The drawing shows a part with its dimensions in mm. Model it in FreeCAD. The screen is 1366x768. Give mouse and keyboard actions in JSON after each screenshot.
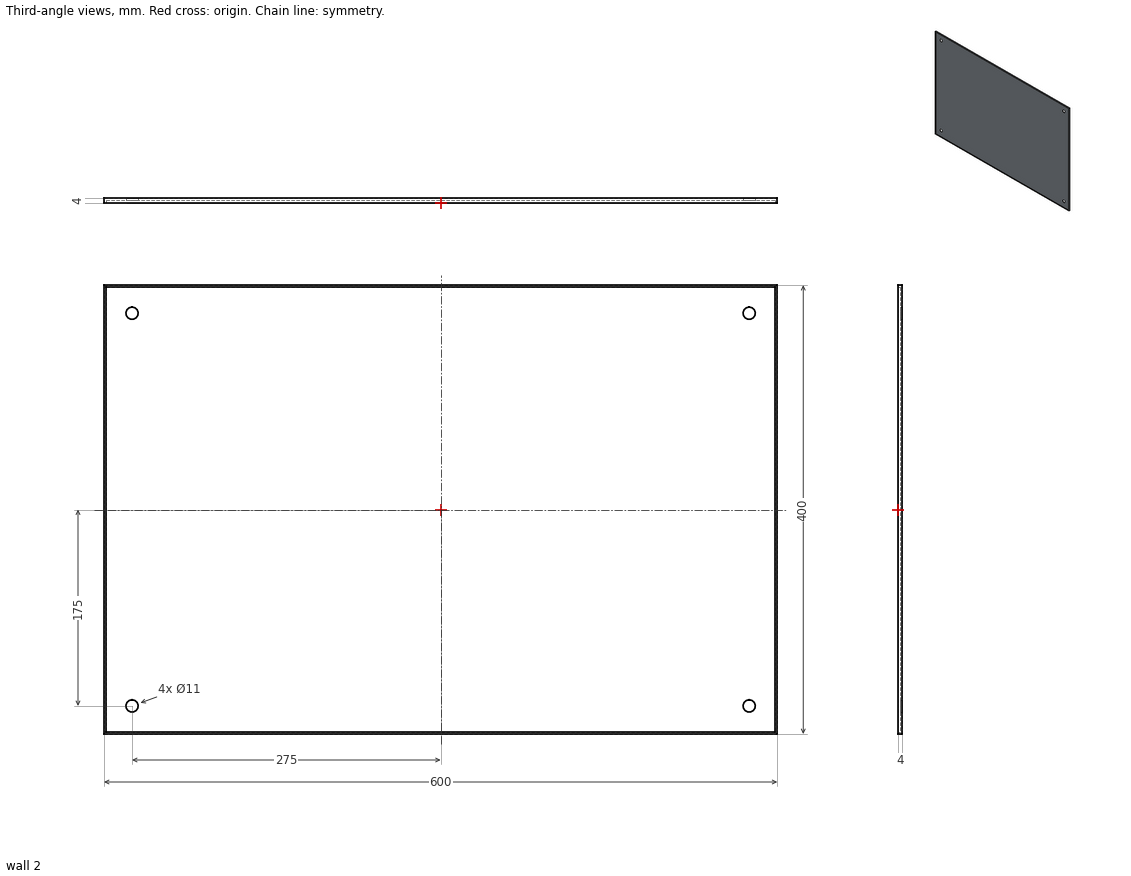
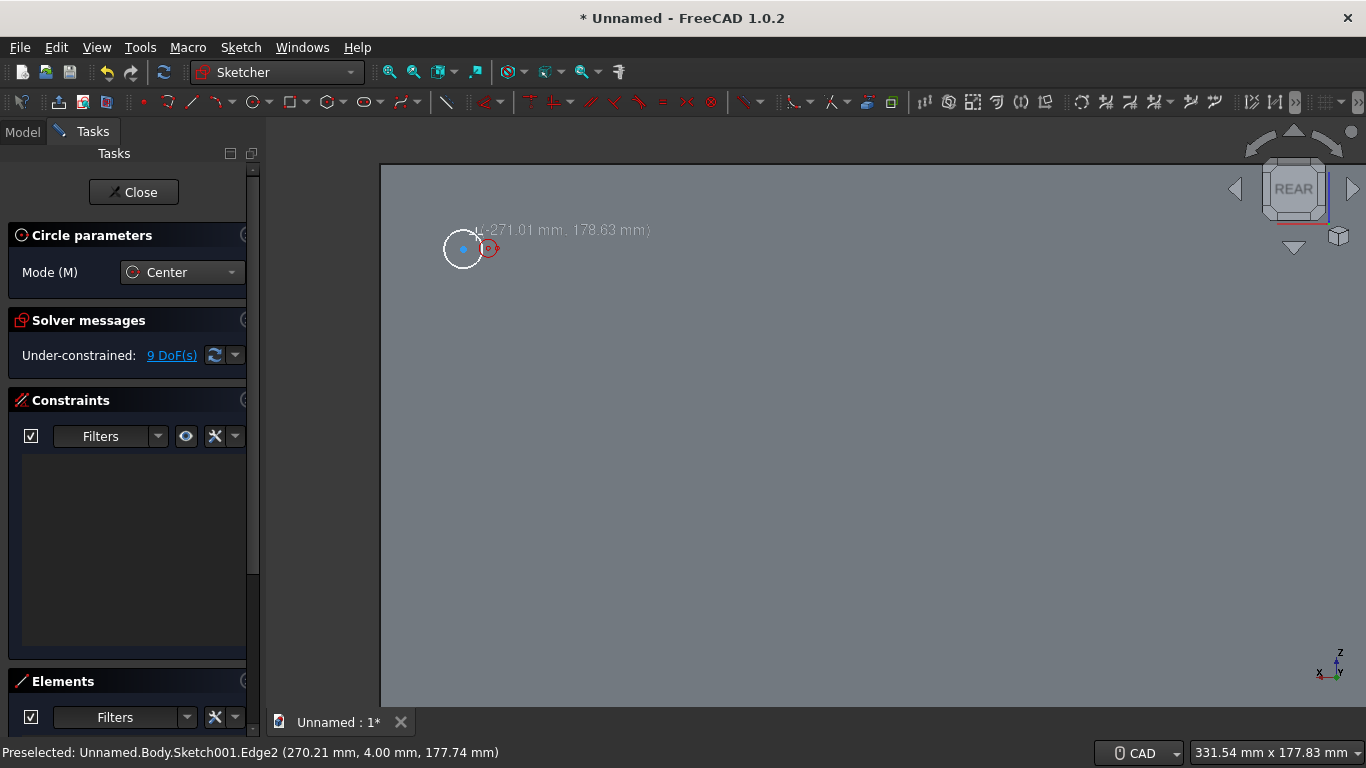
{"action": "scroll", "coordinate": [477, 233], "scroll_direction": "down", "scroll_amount": 6}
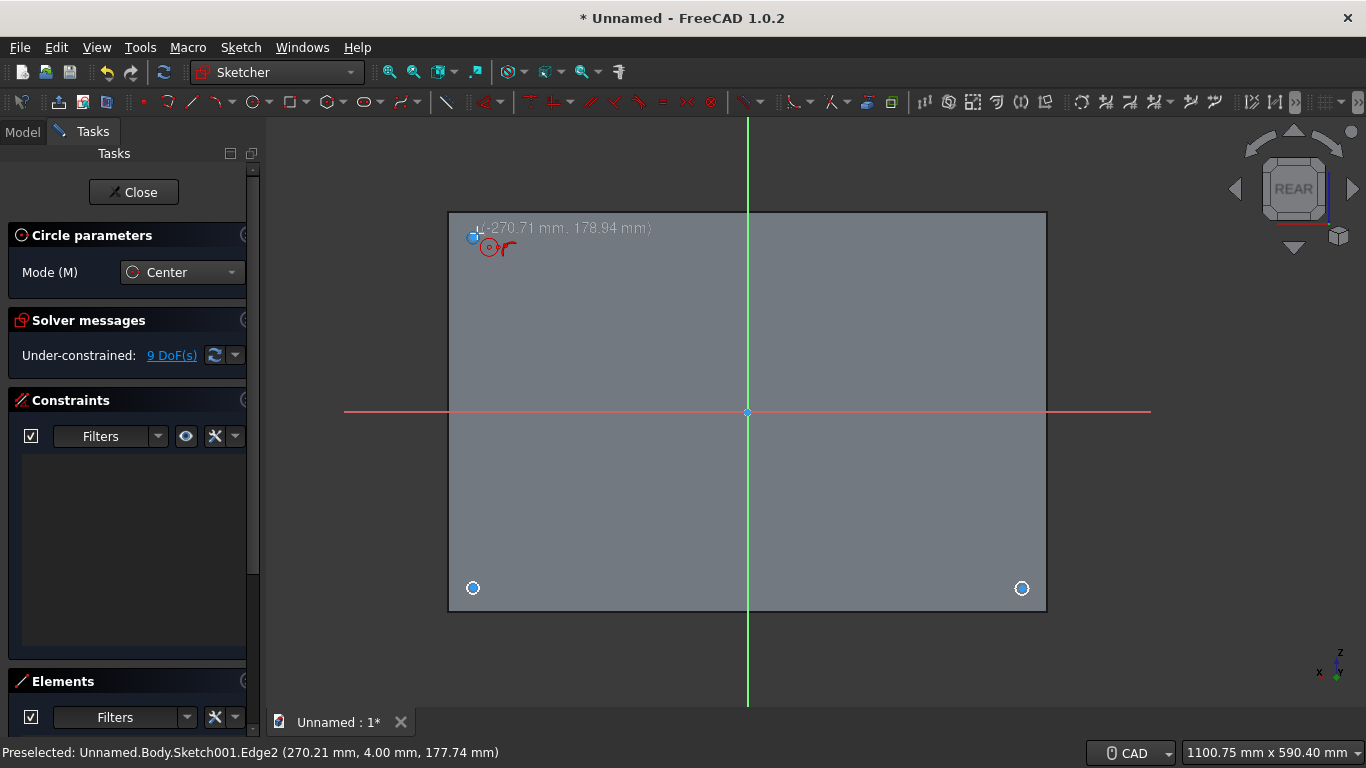
{"action": "scroll", "coordinate": [1022, 237], "scroll_direction": "up", "scroll_amount": 8}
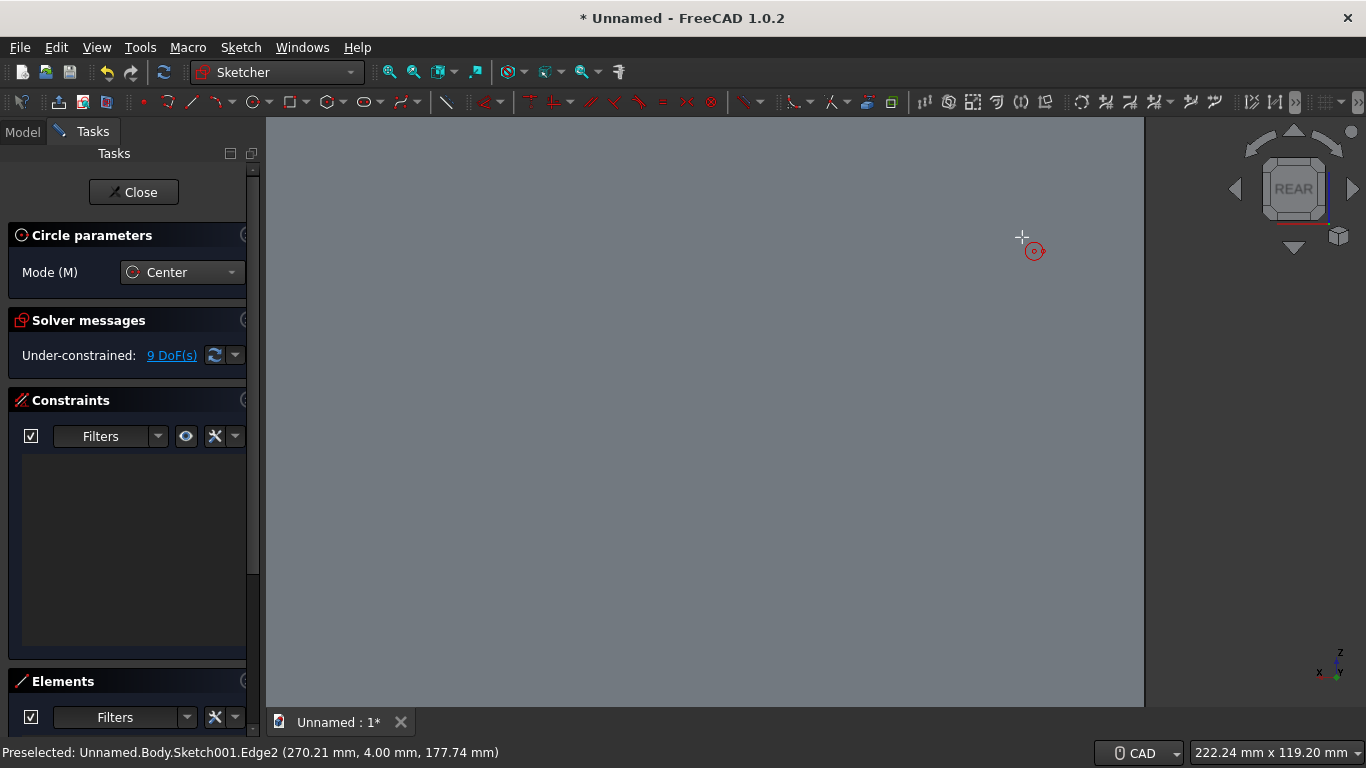
{"action": "scroll", "coordinate": [1022, 237], "scroll_direction": "down", "scroll_amount": 8}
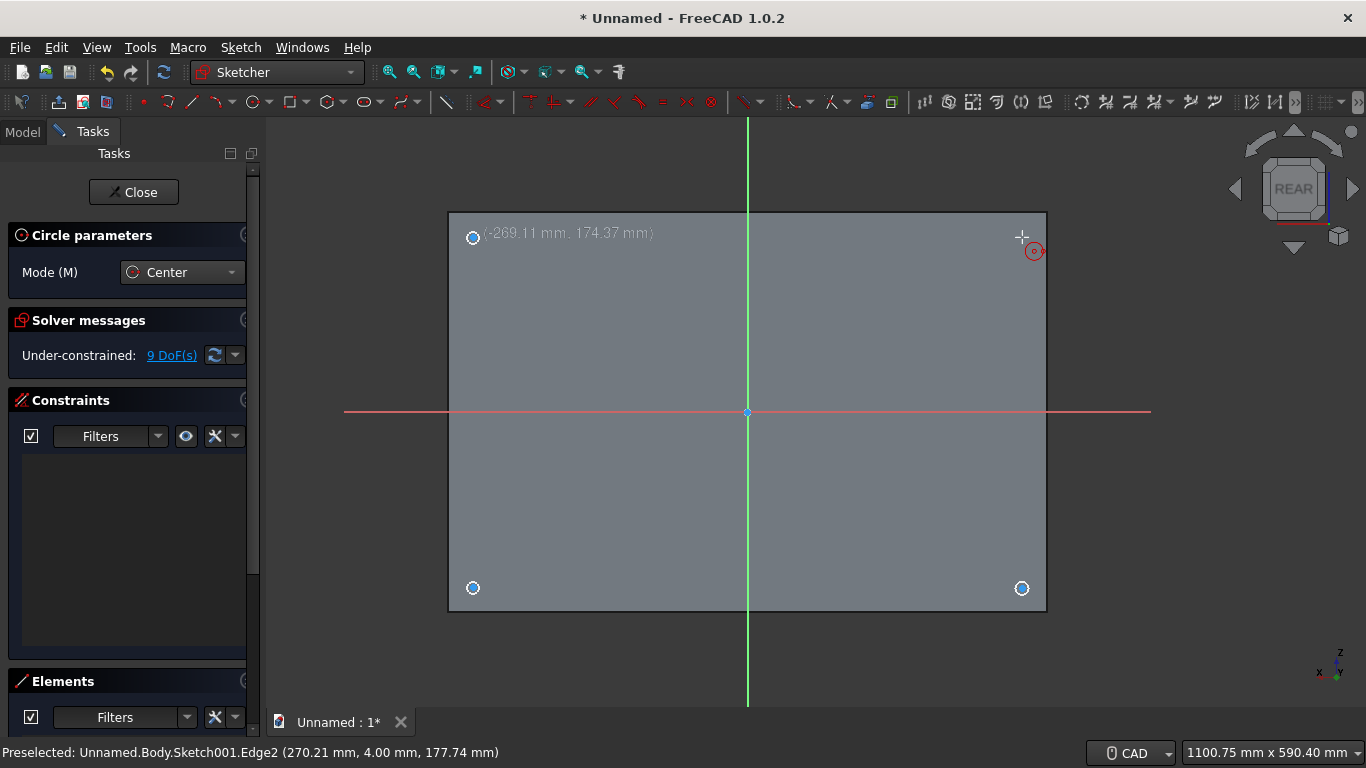
{"action": "left_click", "coordinate": [1022, 237]}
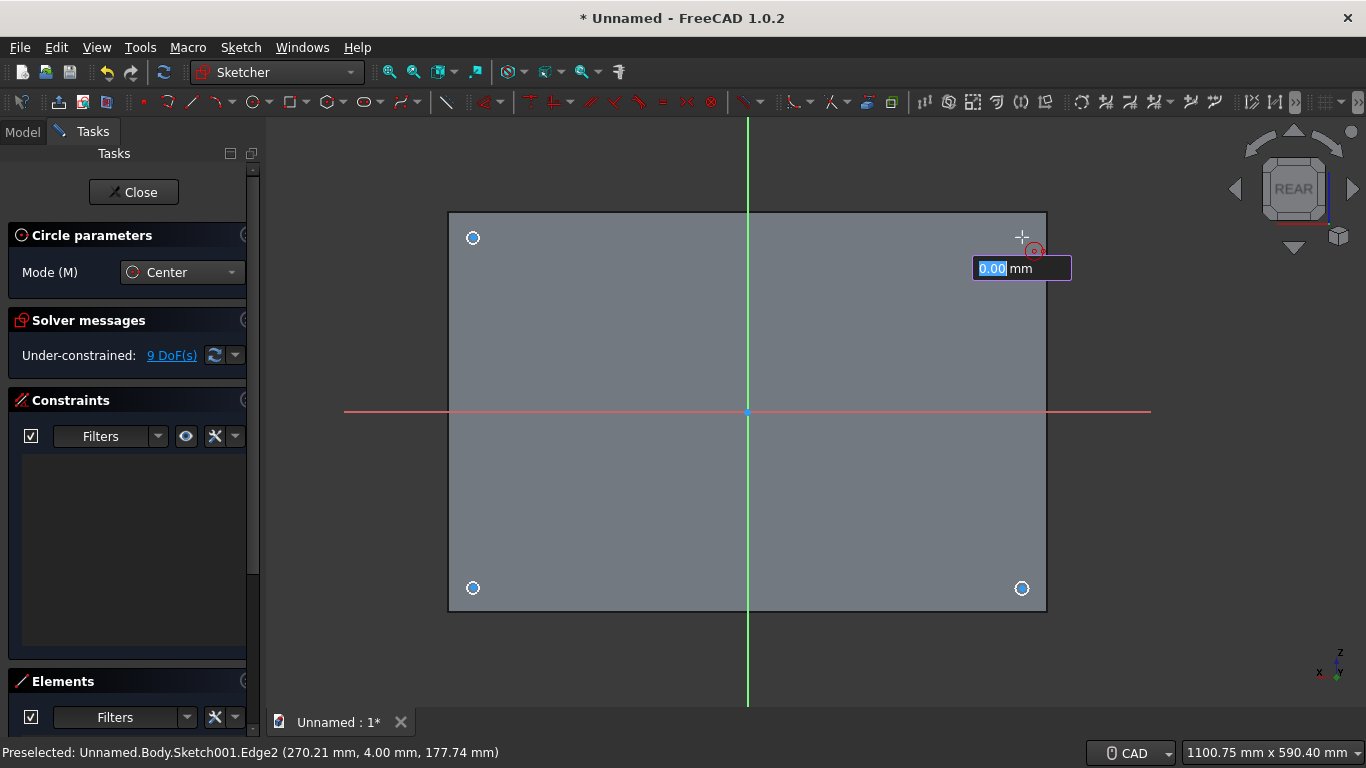
{"action": "scroll", "coordinate": [1026, 233], "scroll_direction": "up", "scroll_amount": 6}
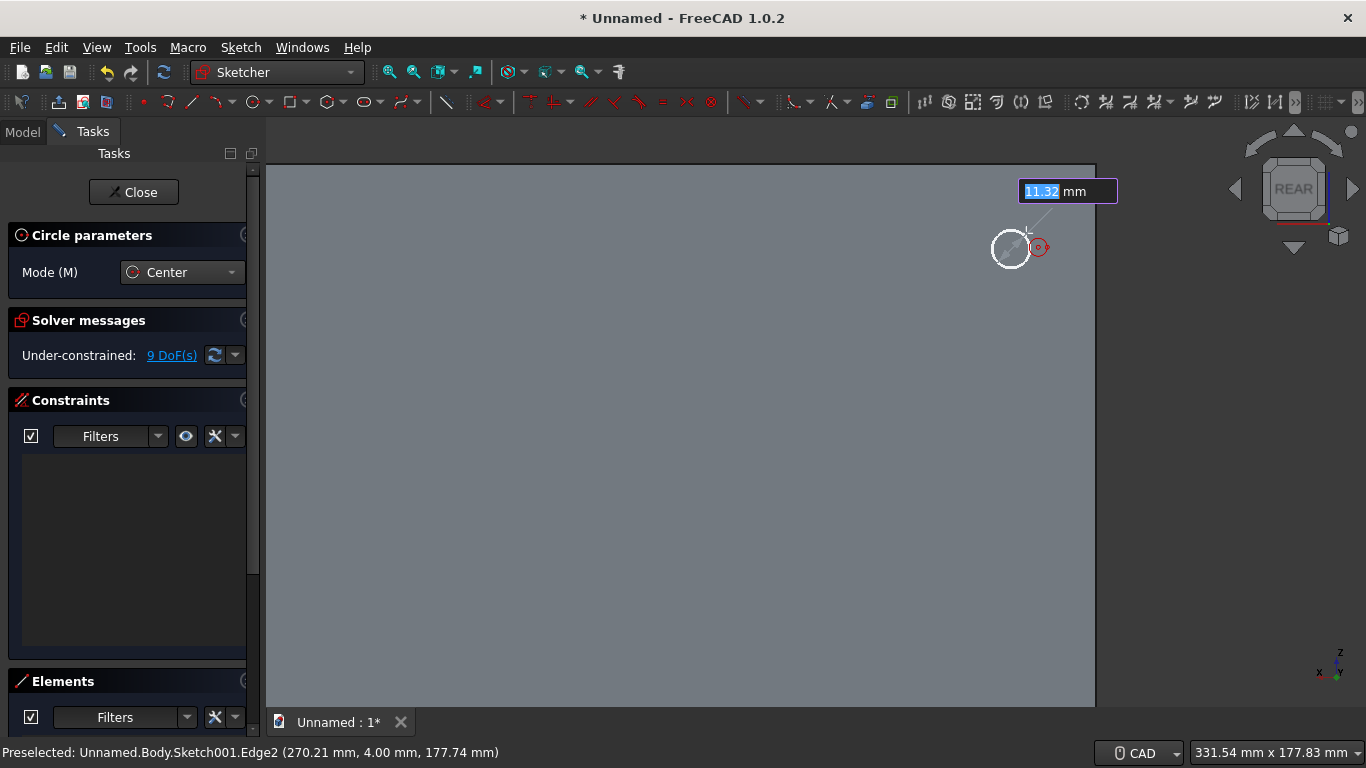
{"action": "left_click", "coordinate": [1026, 234]}
{"action": "key", "text": "Escape"}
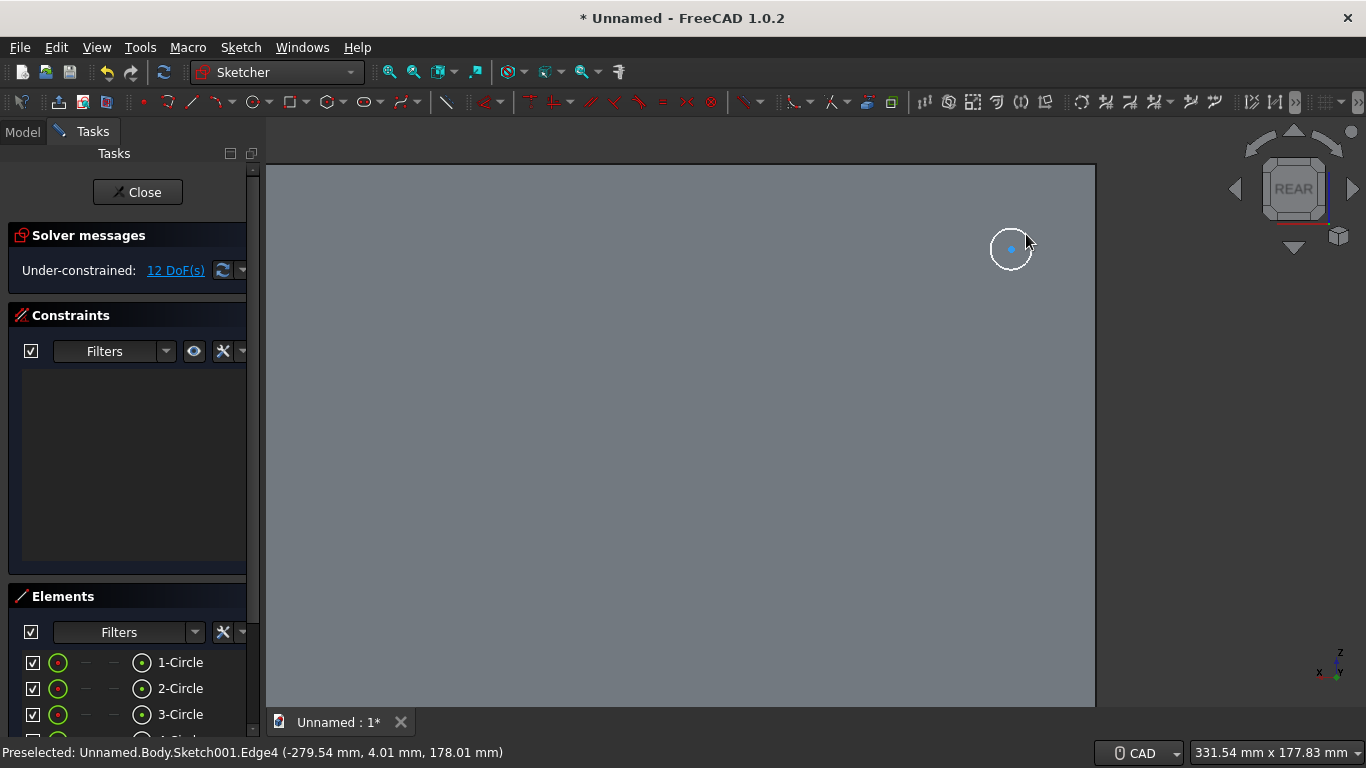
{"action": "scroll", "coordinate": [1026, 233], "scroll_direction": "down", "scroll_amount": 6}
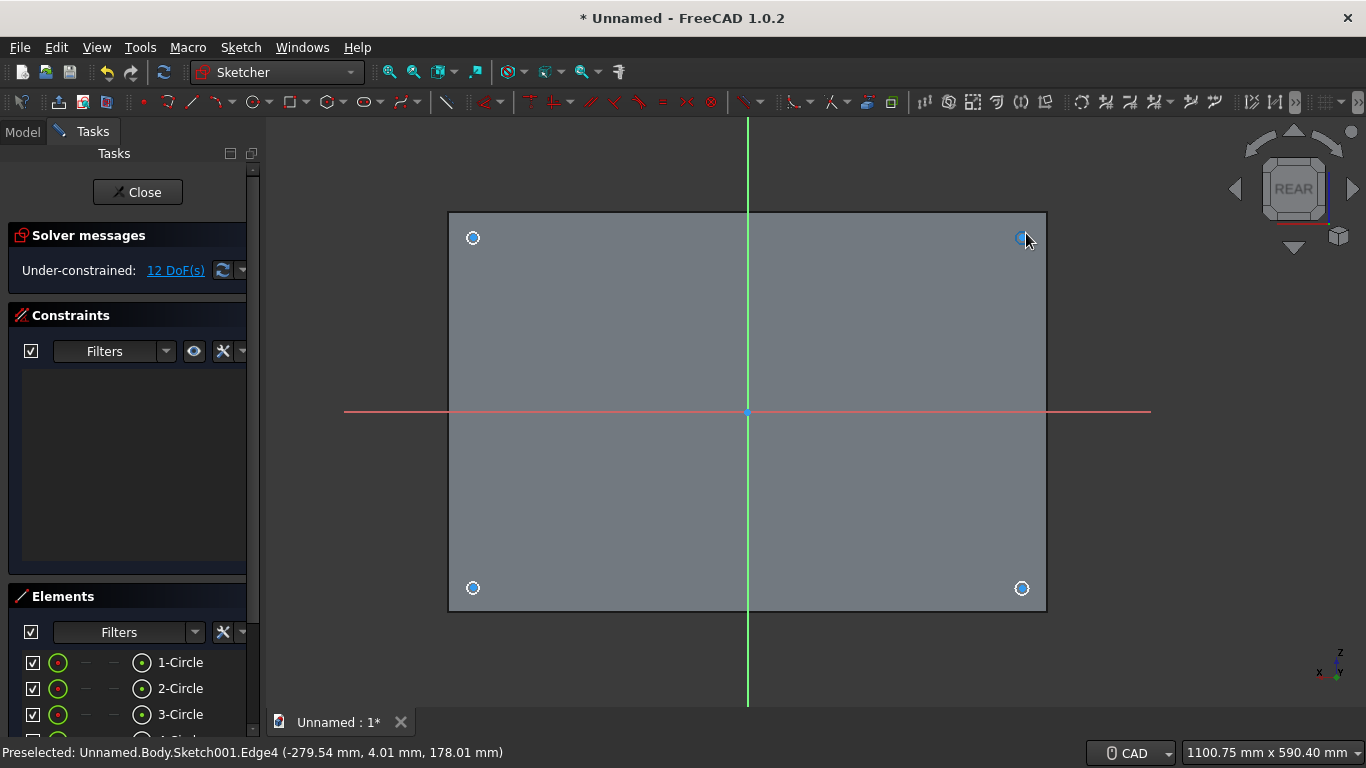
{"action": "scroll", "coordinate": [1027, 584], "scroll_direction": "up", "scroll_amount": 4}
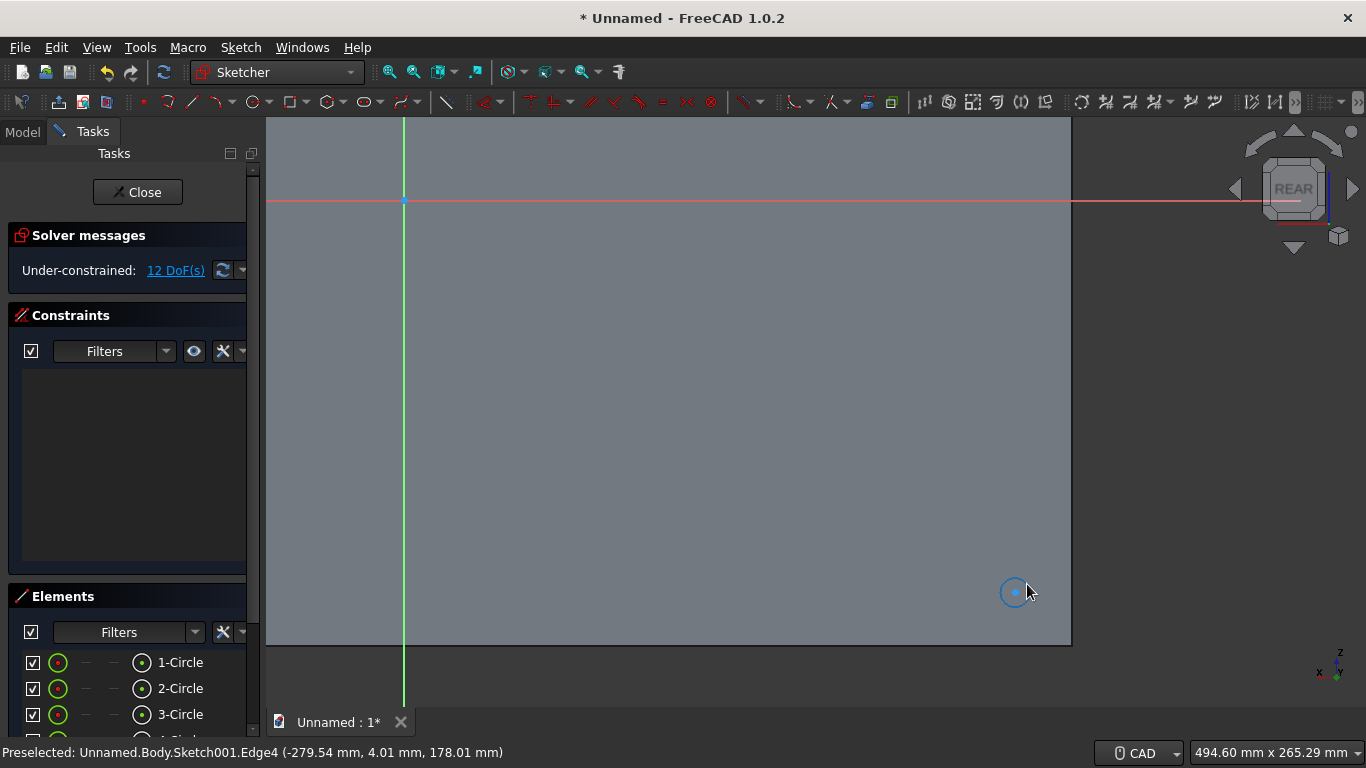
{"action": "left_click", "coordinate": [1025, 582]}